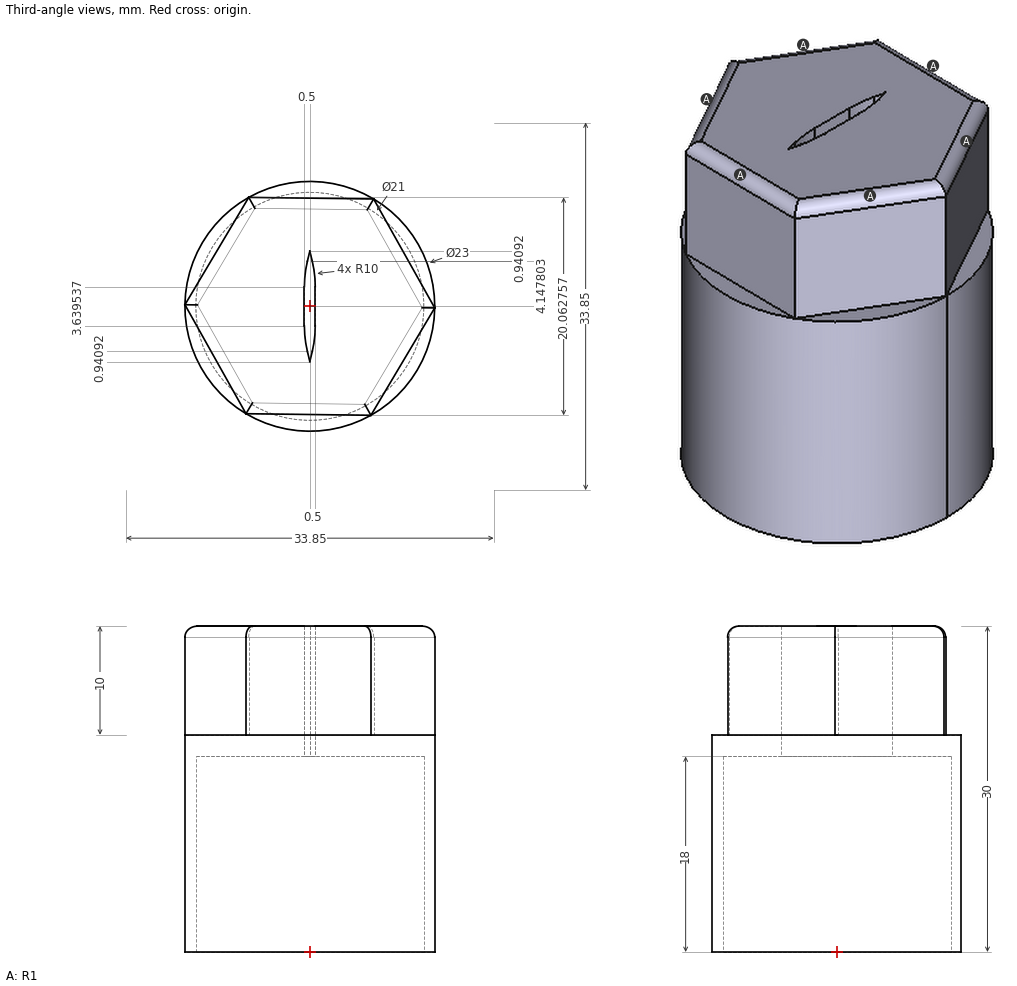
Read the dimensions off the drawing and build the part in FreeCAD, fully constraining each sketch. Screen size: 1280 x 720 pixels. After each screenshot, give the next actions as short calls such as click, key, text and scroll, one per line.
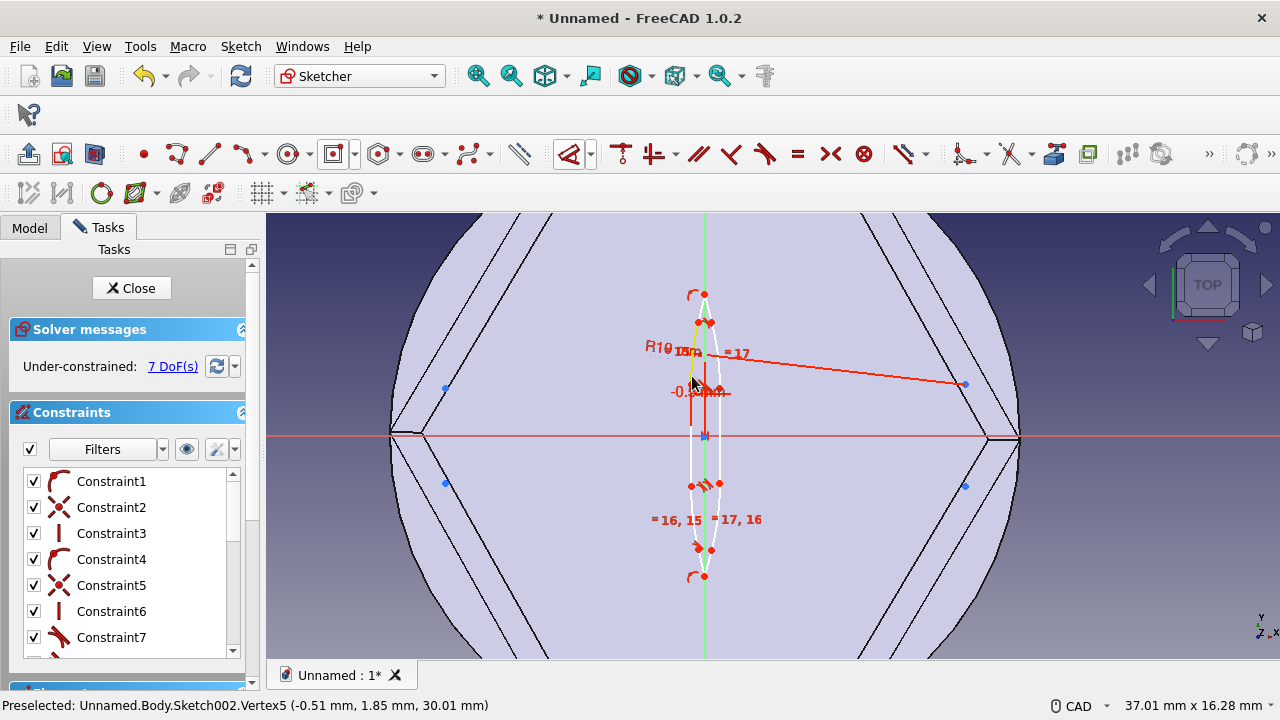
scroll(720, 483, up, 6)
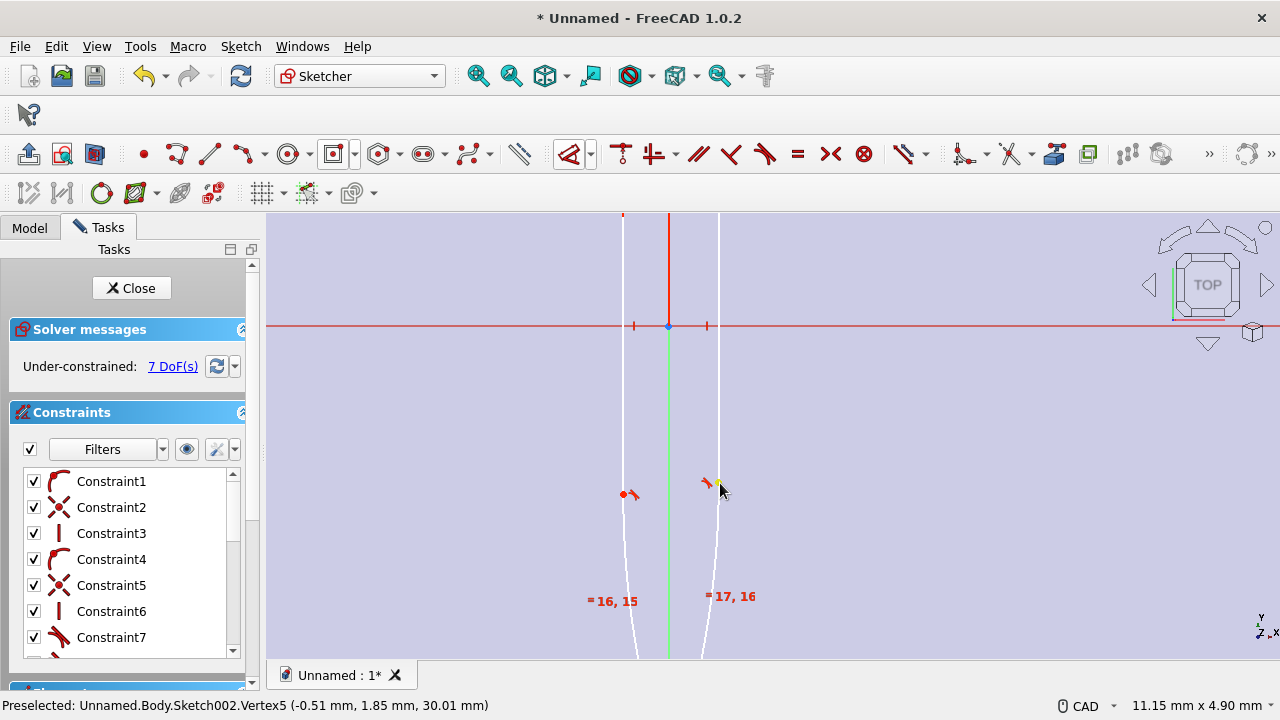
click(719, 482)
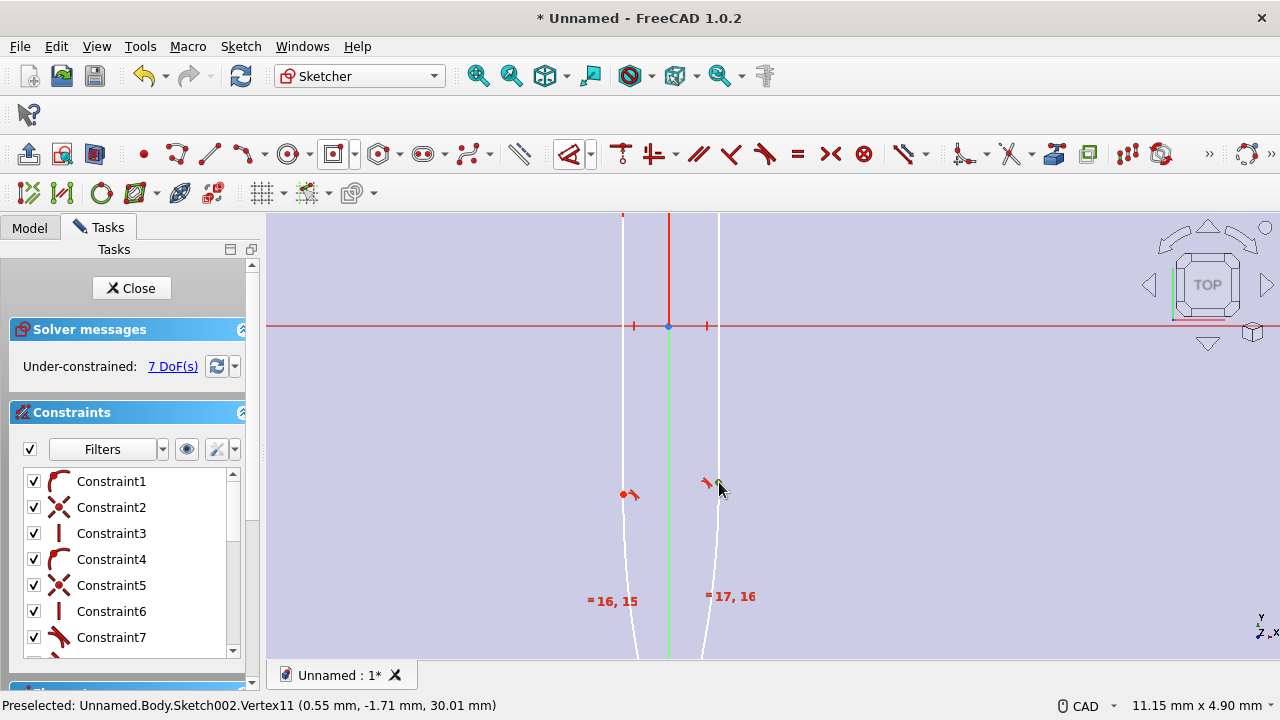
click(590, 154)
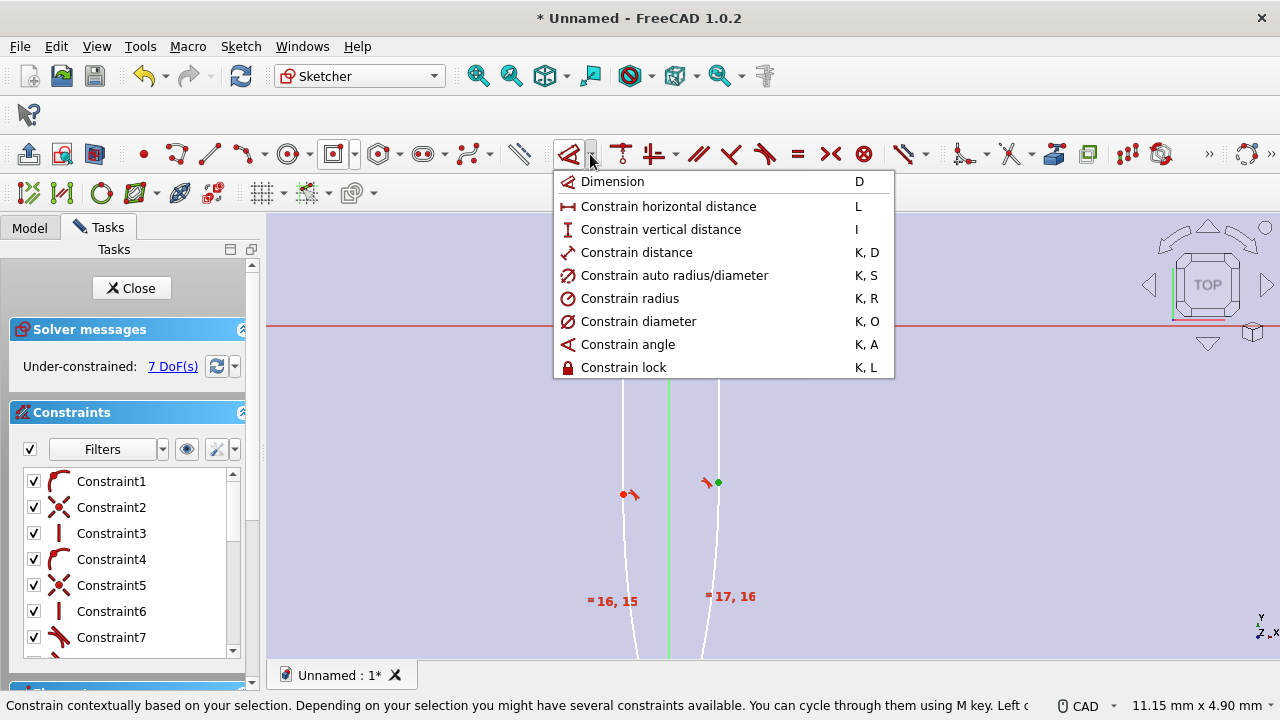
click(724, 206)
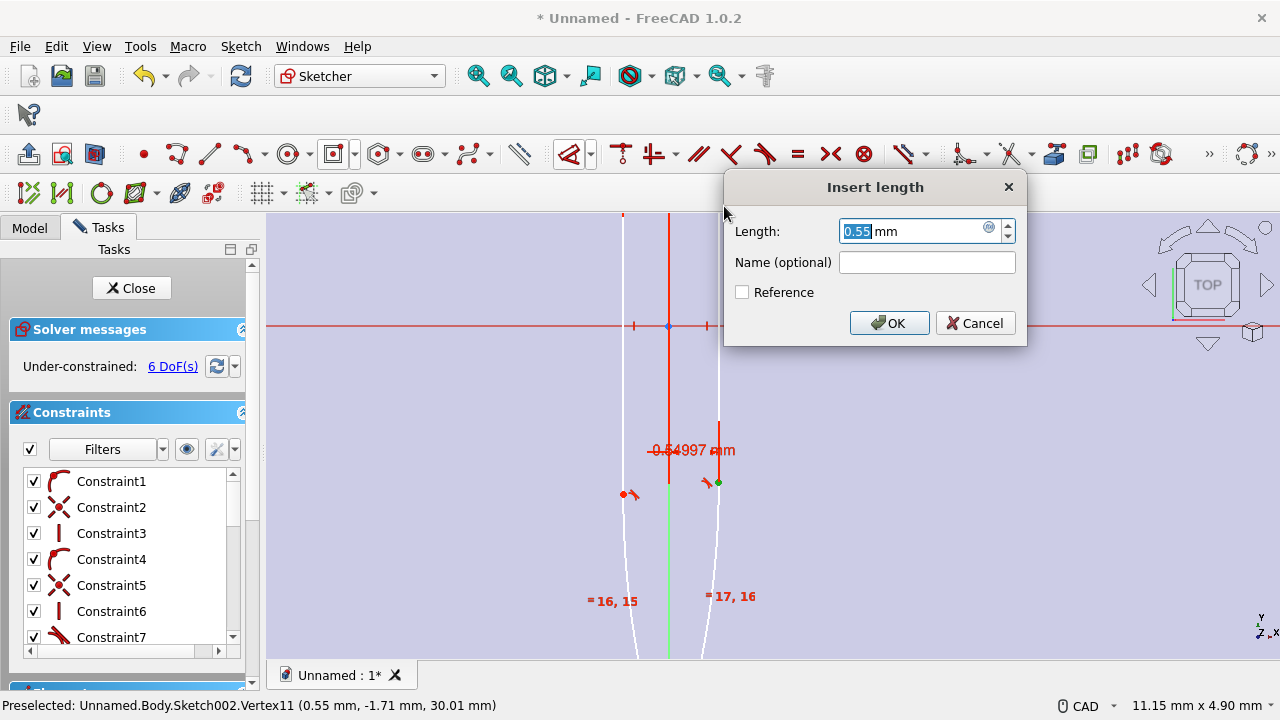
text(0.5)
key(Return)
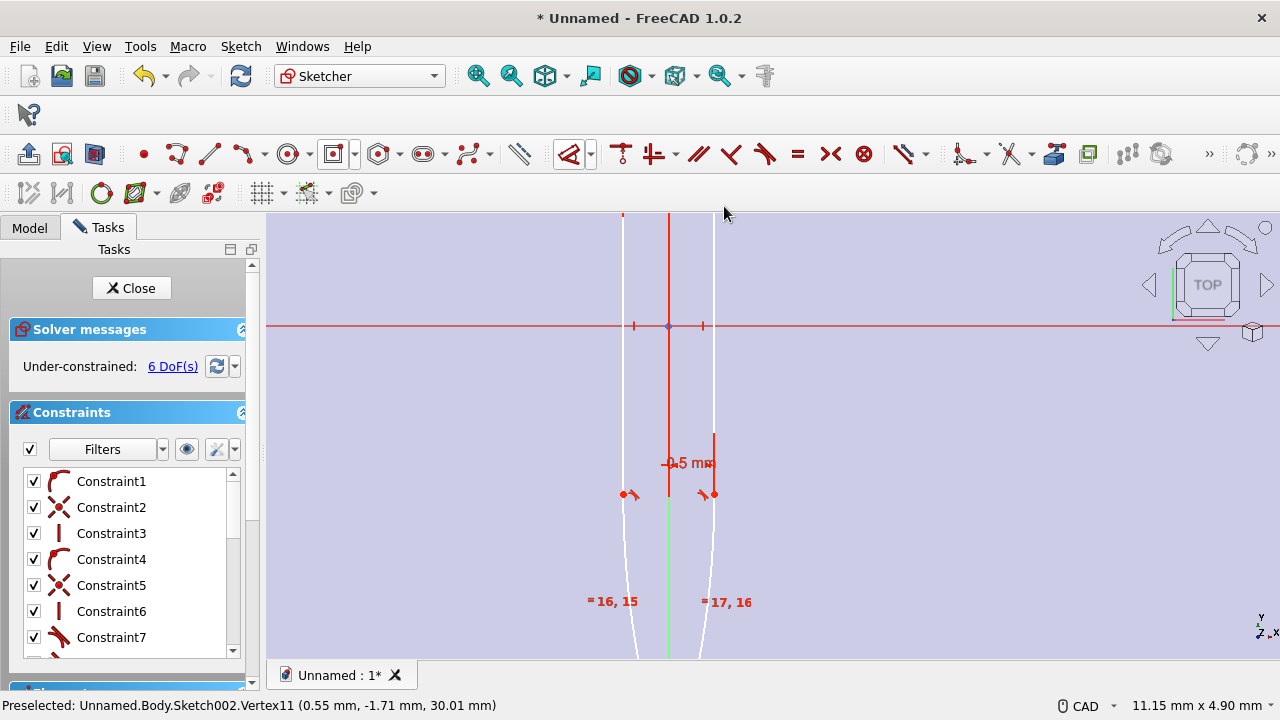
click(623, 257)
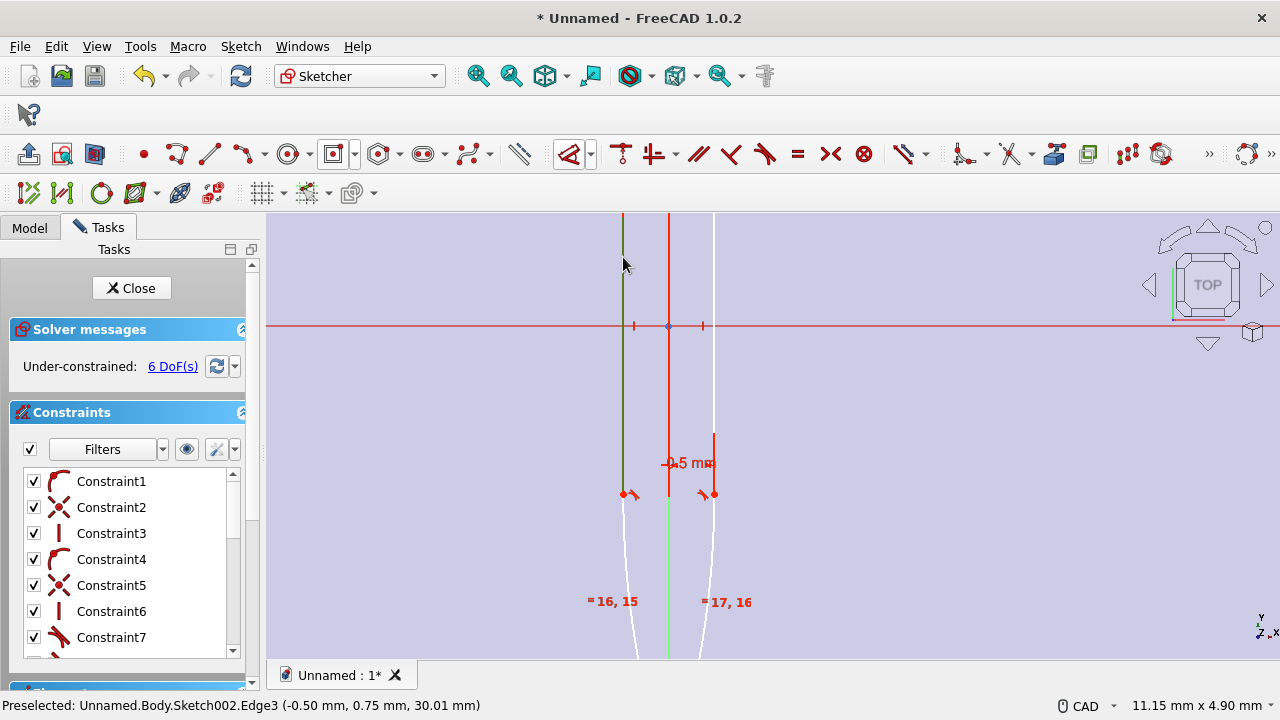
click(590, 154)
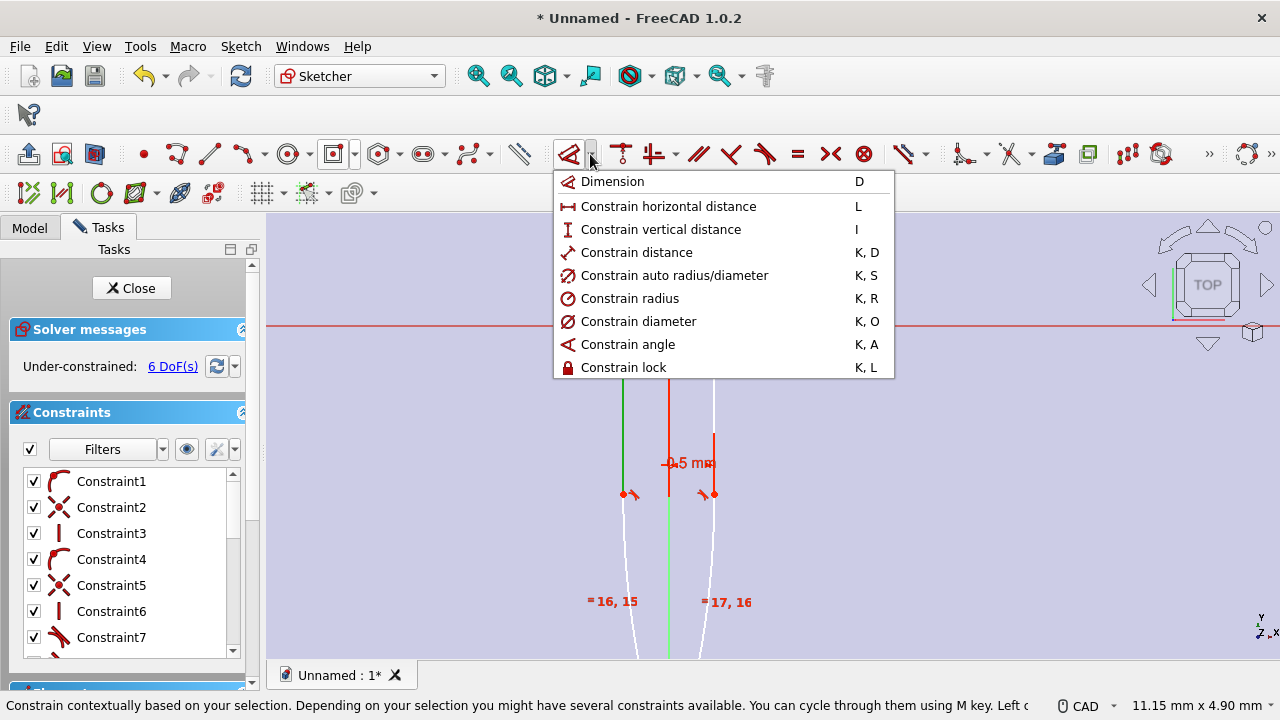
click(724, 230)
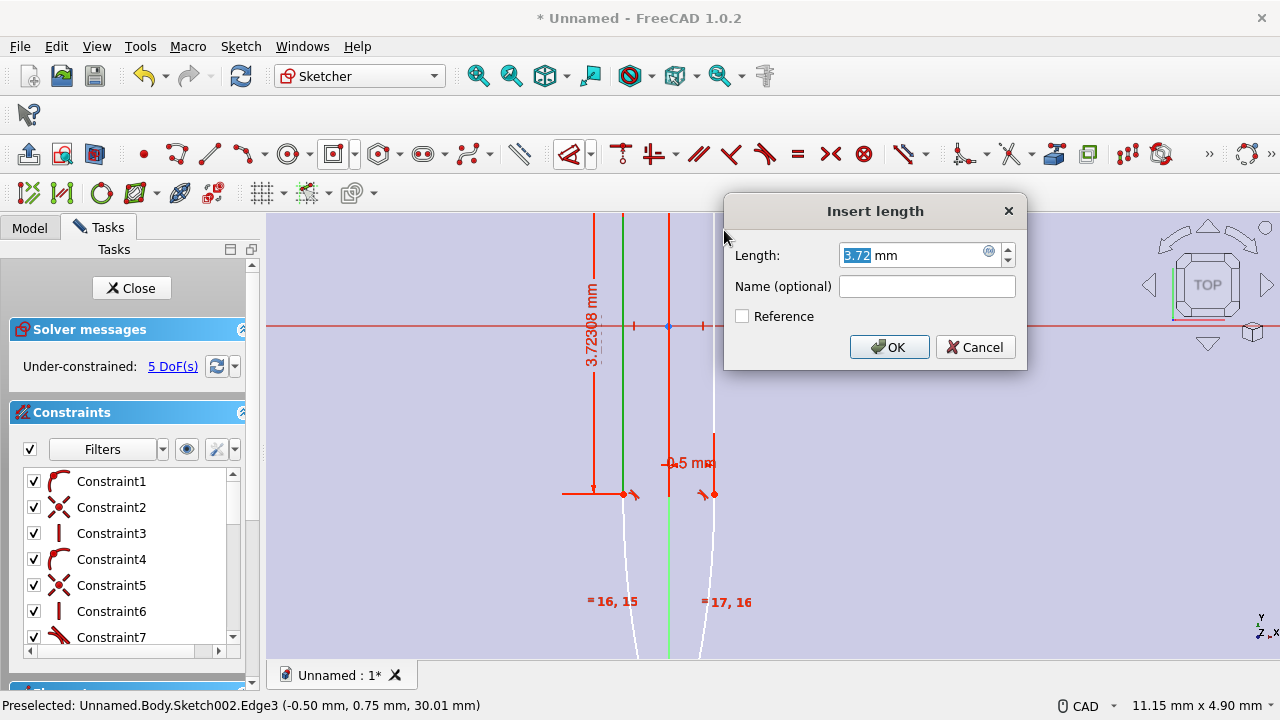
text(3.639537)
key(Return)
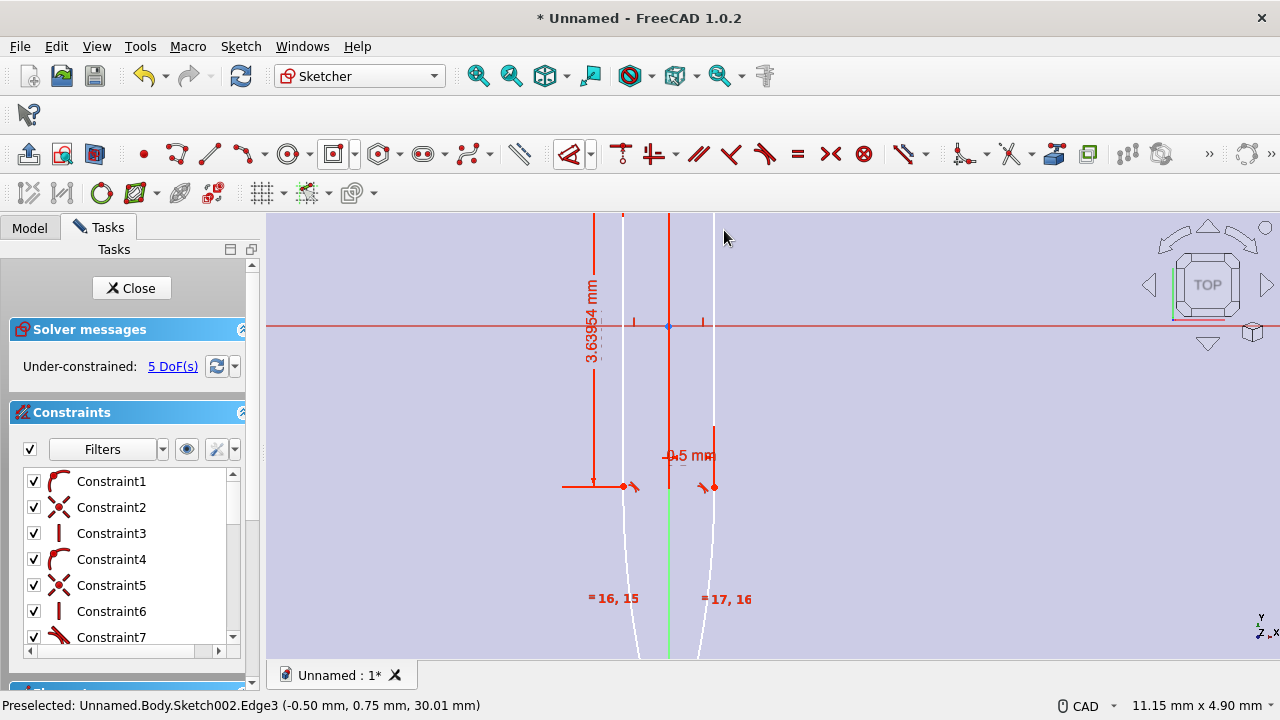
click(714, 388)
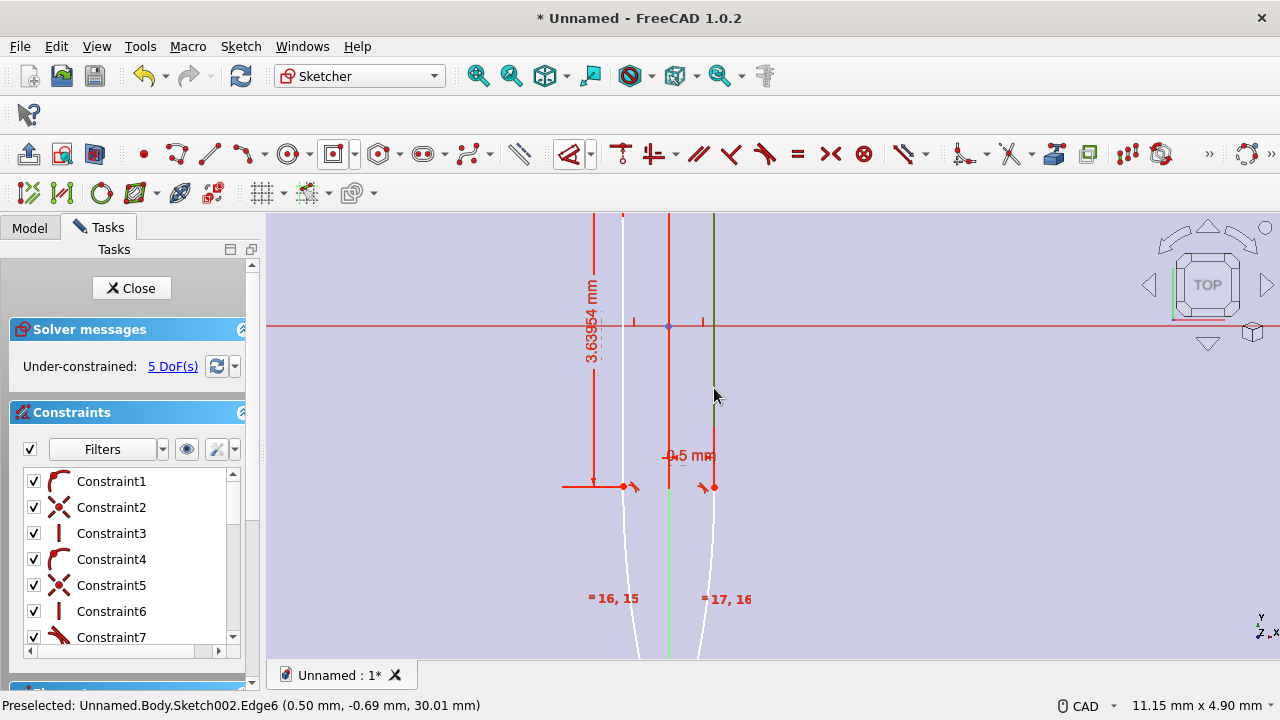
click(590, 154)